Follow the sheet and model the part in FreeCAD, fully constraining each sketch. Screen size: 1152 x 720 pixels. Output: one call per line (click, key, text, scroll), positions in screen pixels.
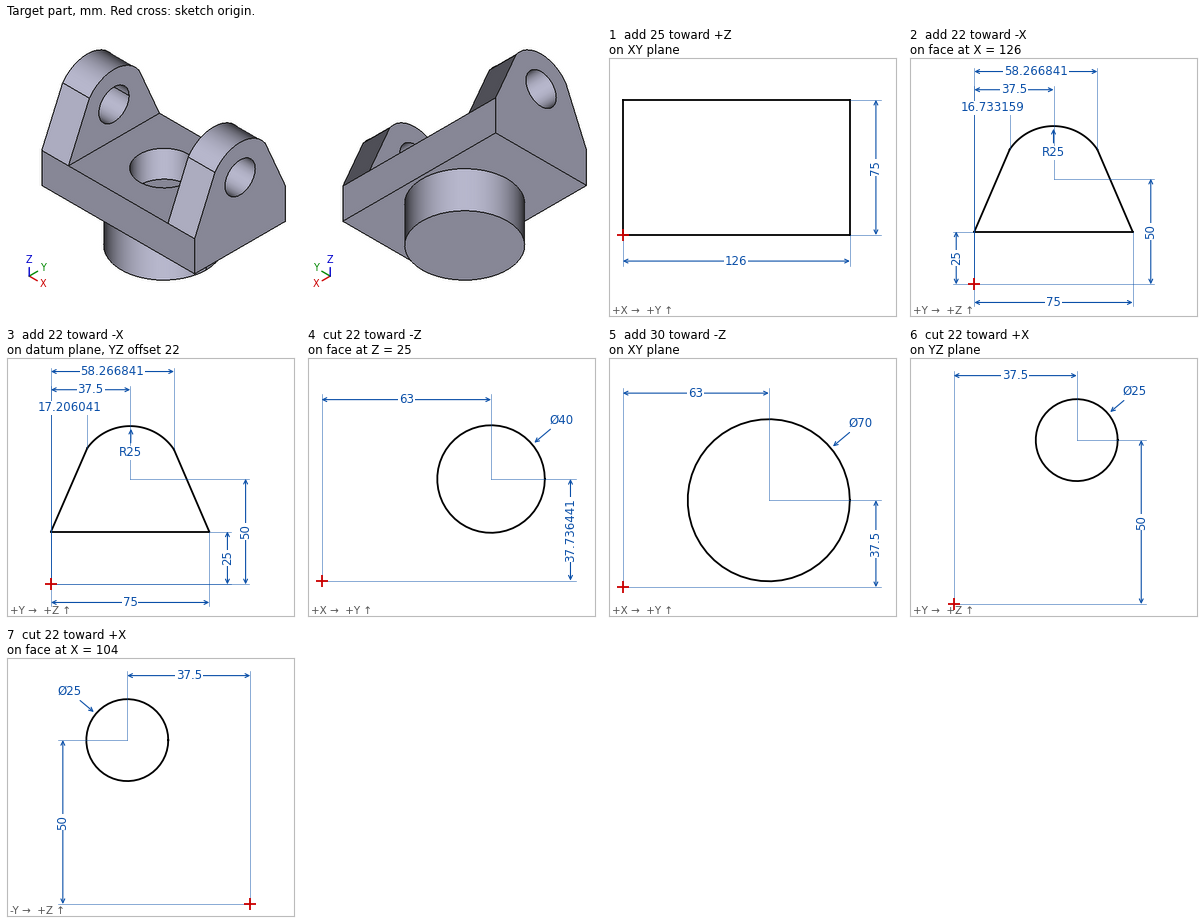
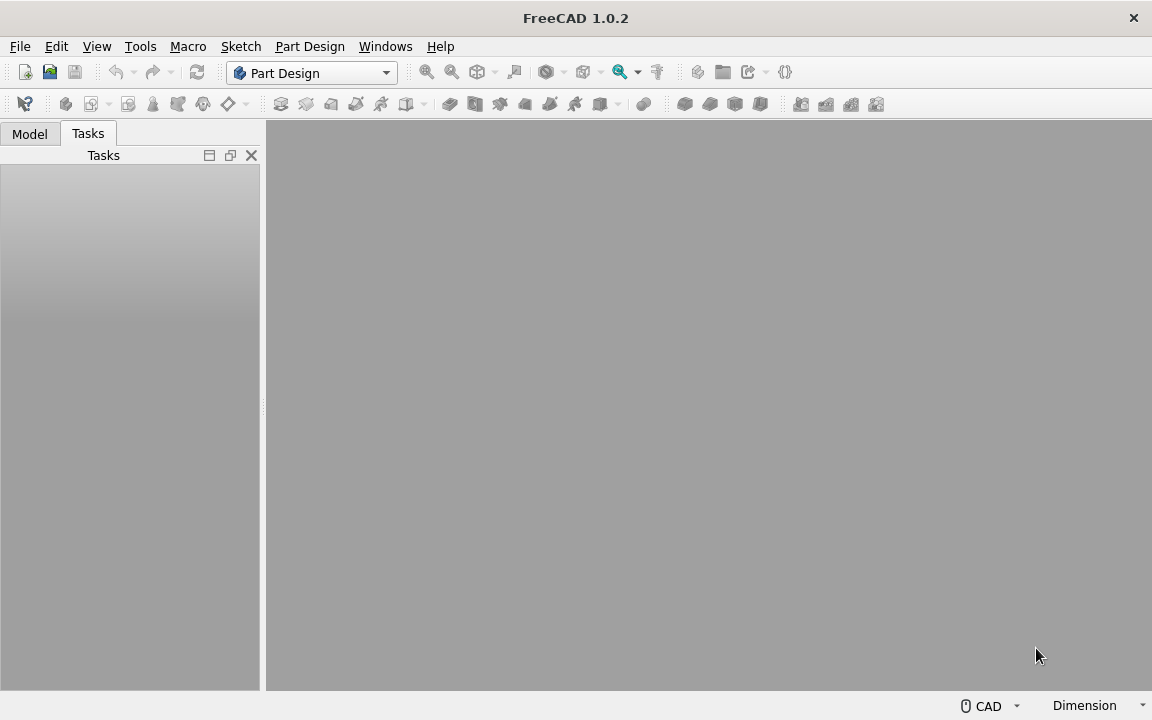
click(25, 72)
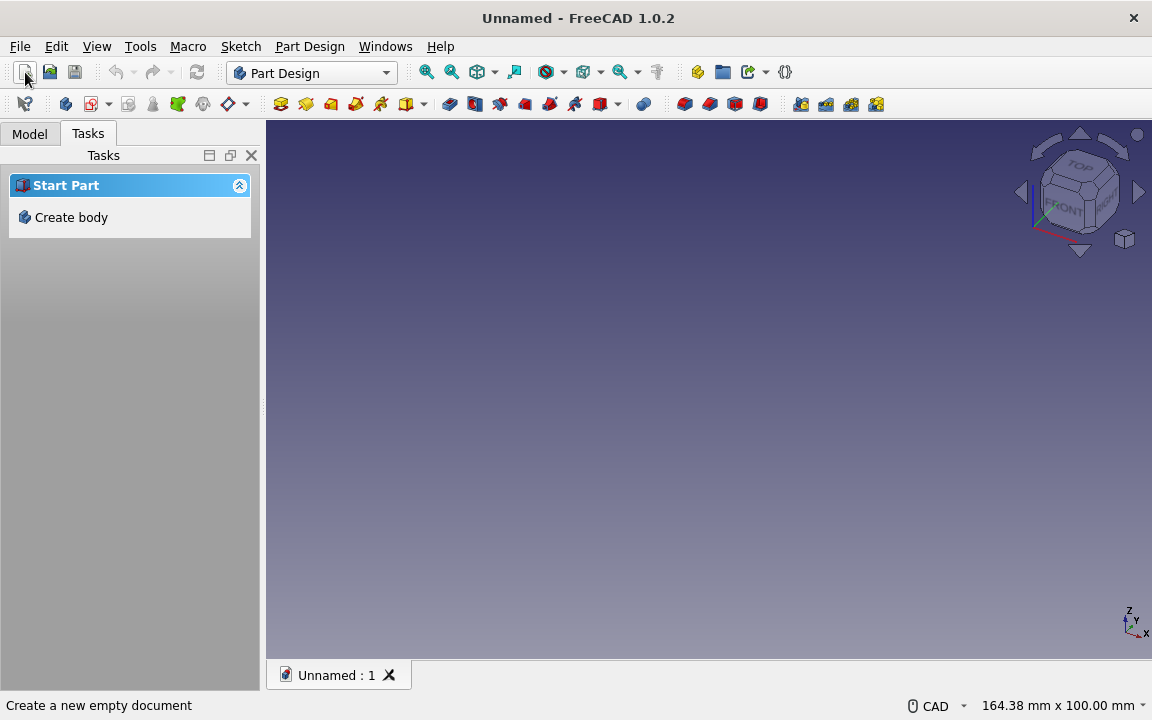
click(90, 104)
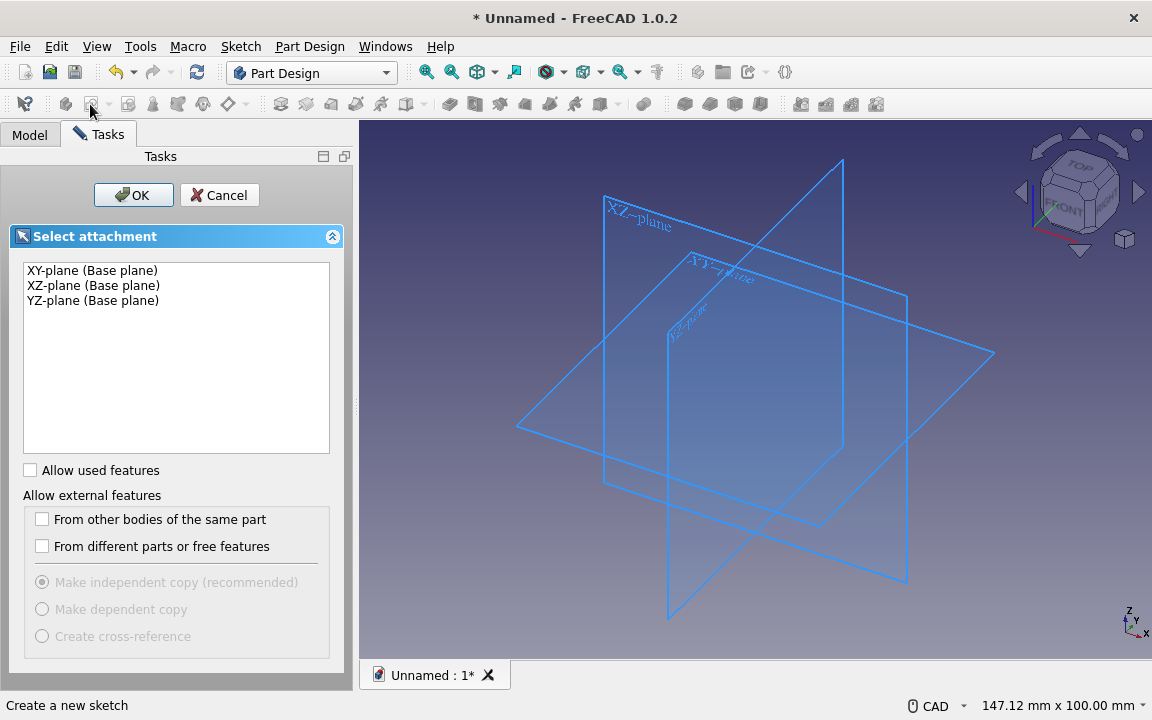
click(84, 270)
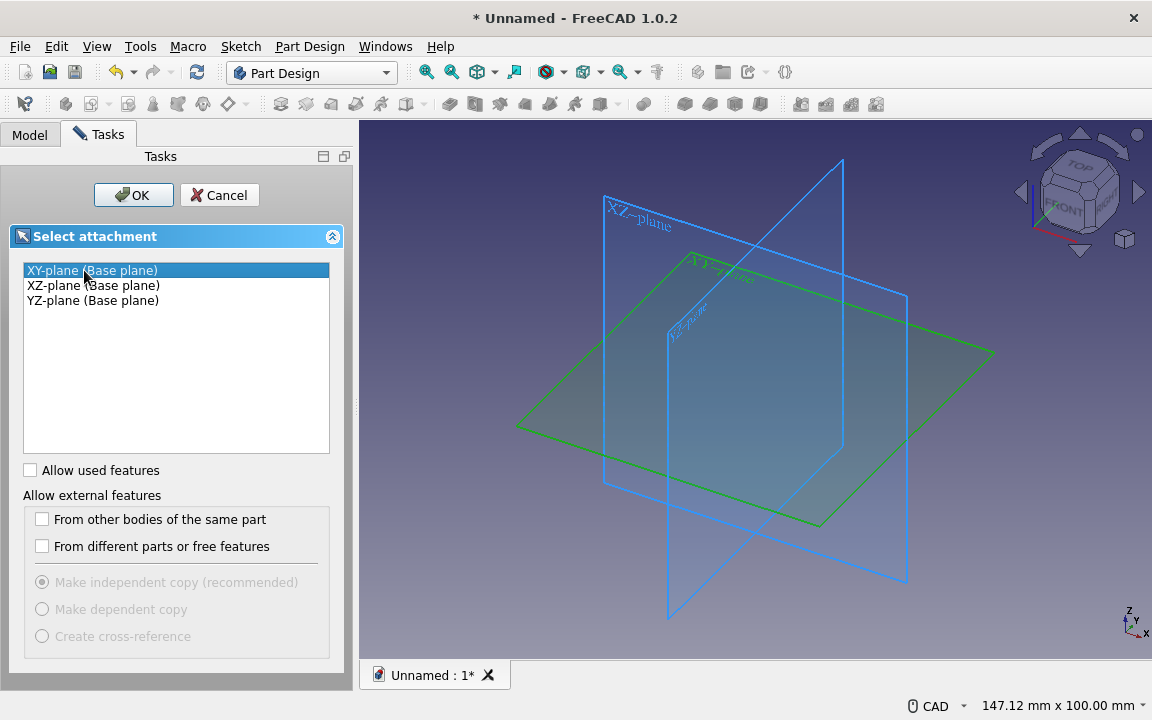
click(134, 195)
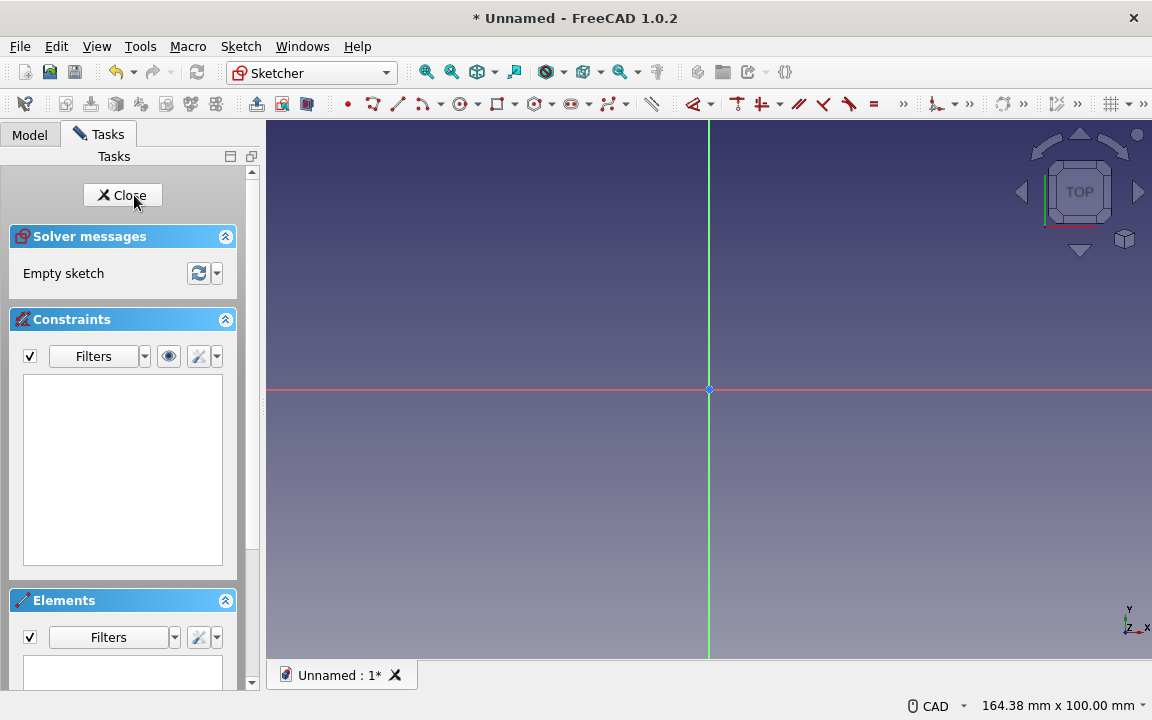
scroll(294, 631, down, 3)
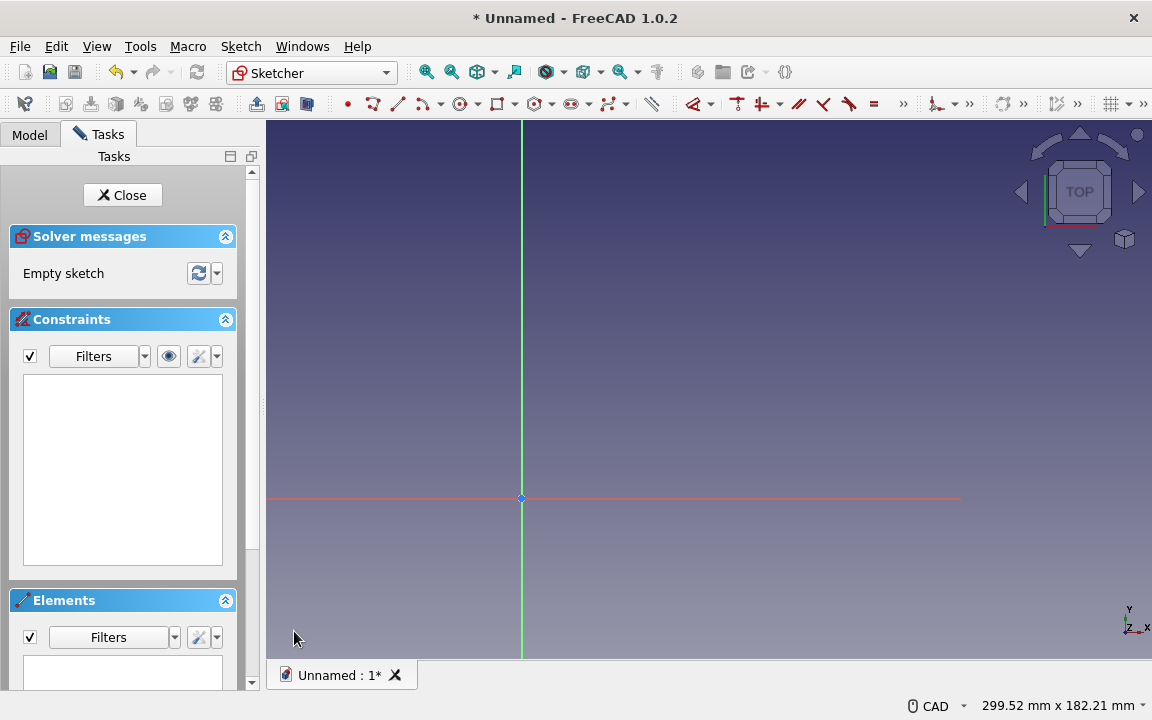
click(496, 104)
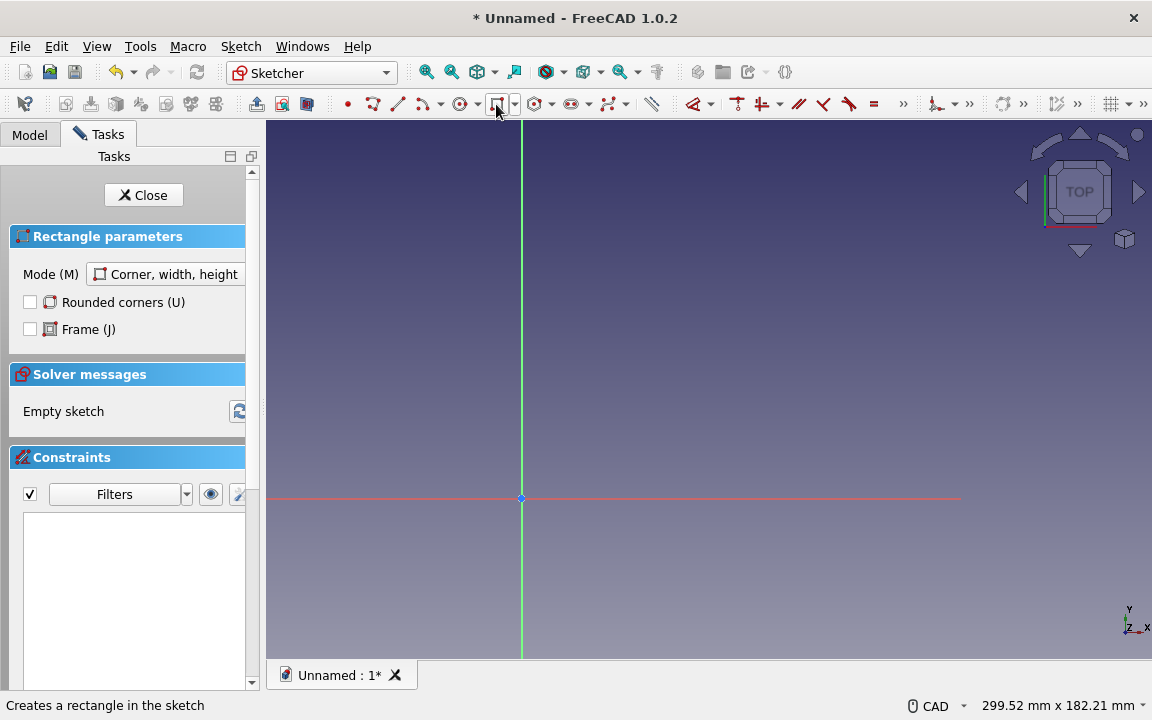
click(522, 499)
move(894, 277)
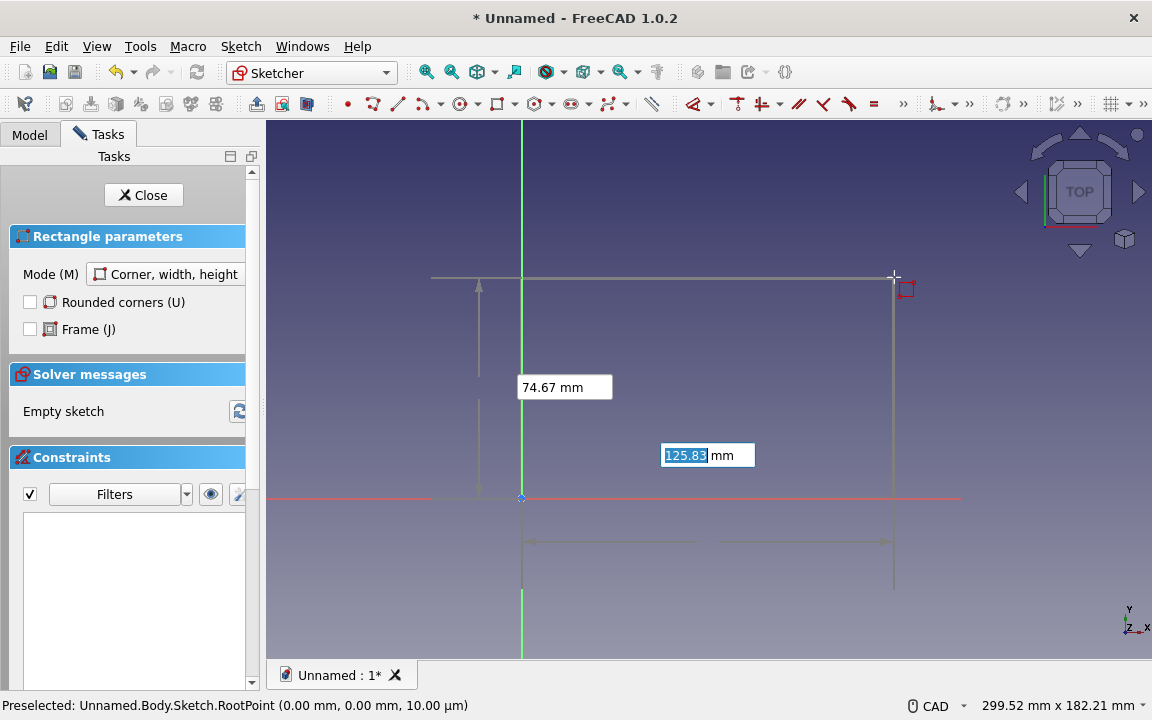
text(126)
key(Tab)
text(75)
key(Return)
key(Escape)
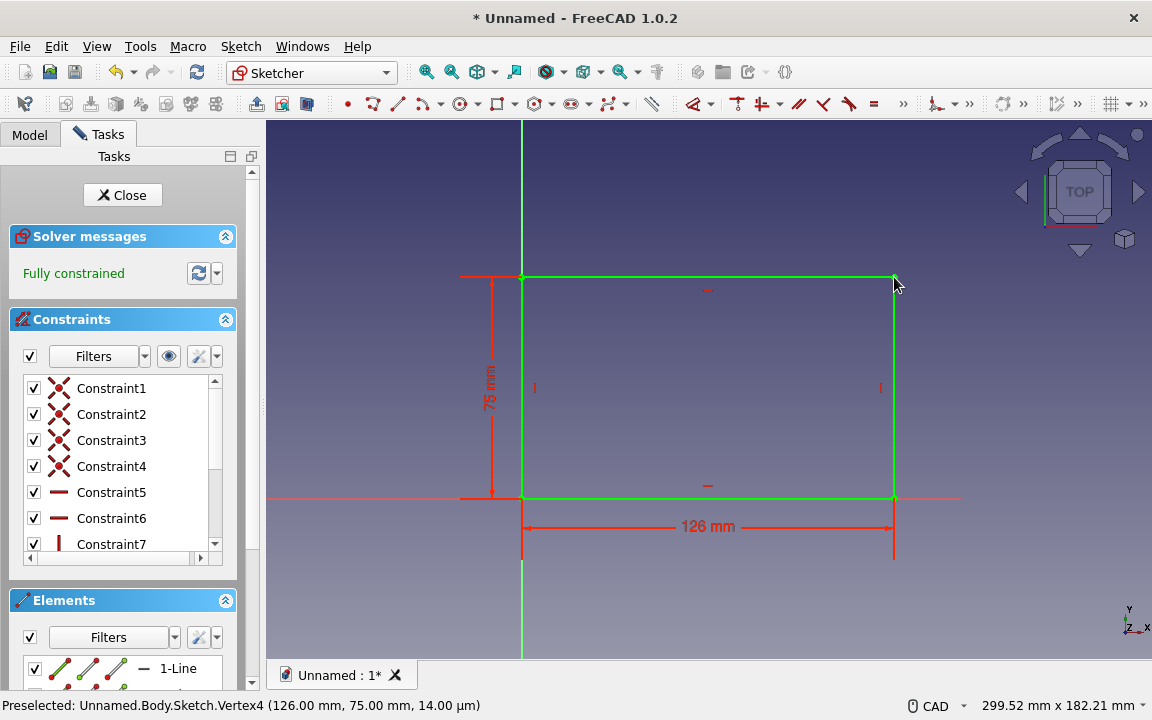
click(123, 195)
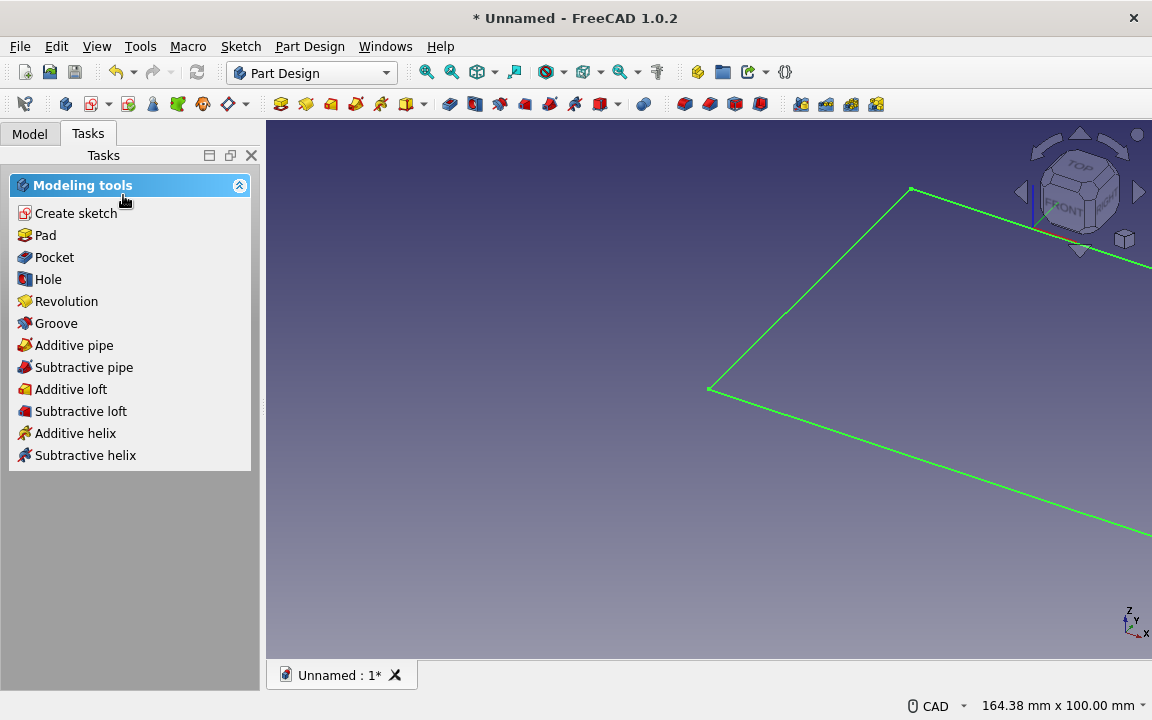
click(281, 104)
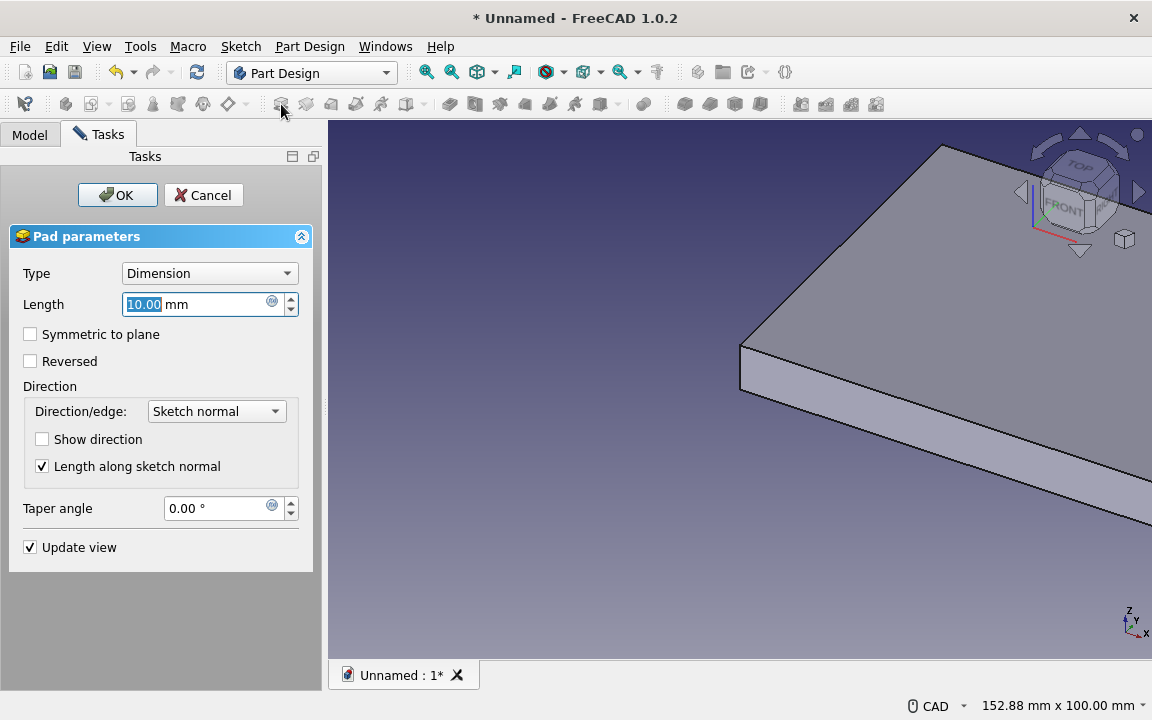
text(25)
key(Tab)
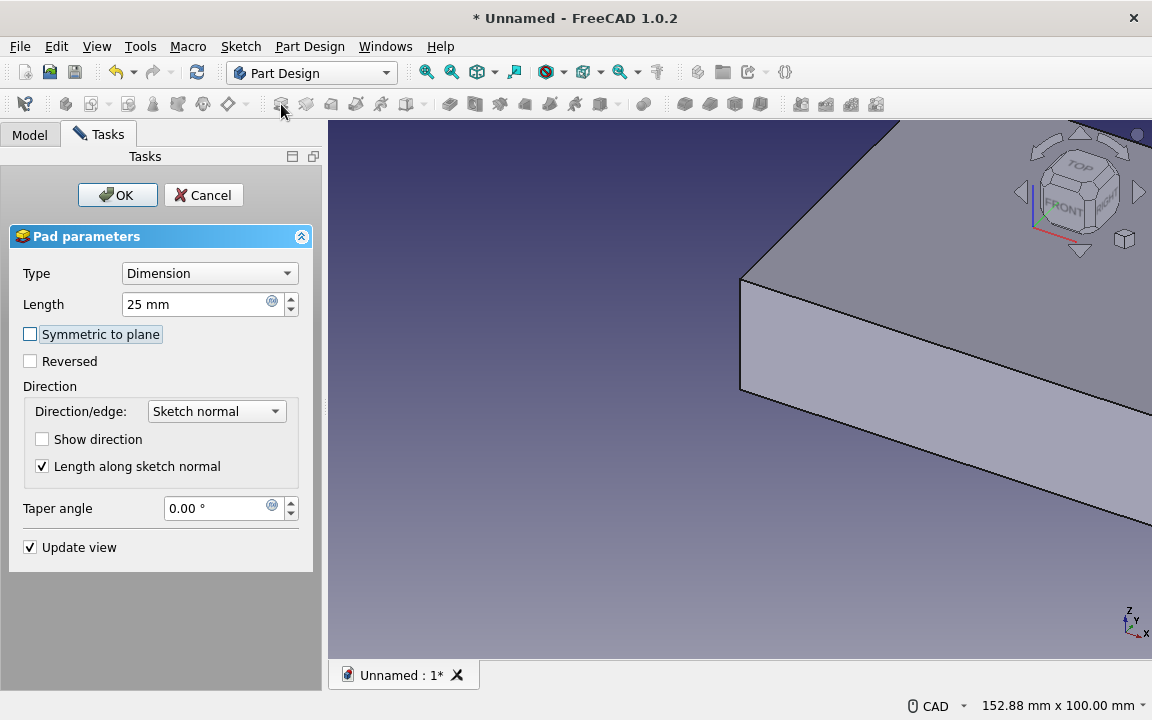
click(118, 195)